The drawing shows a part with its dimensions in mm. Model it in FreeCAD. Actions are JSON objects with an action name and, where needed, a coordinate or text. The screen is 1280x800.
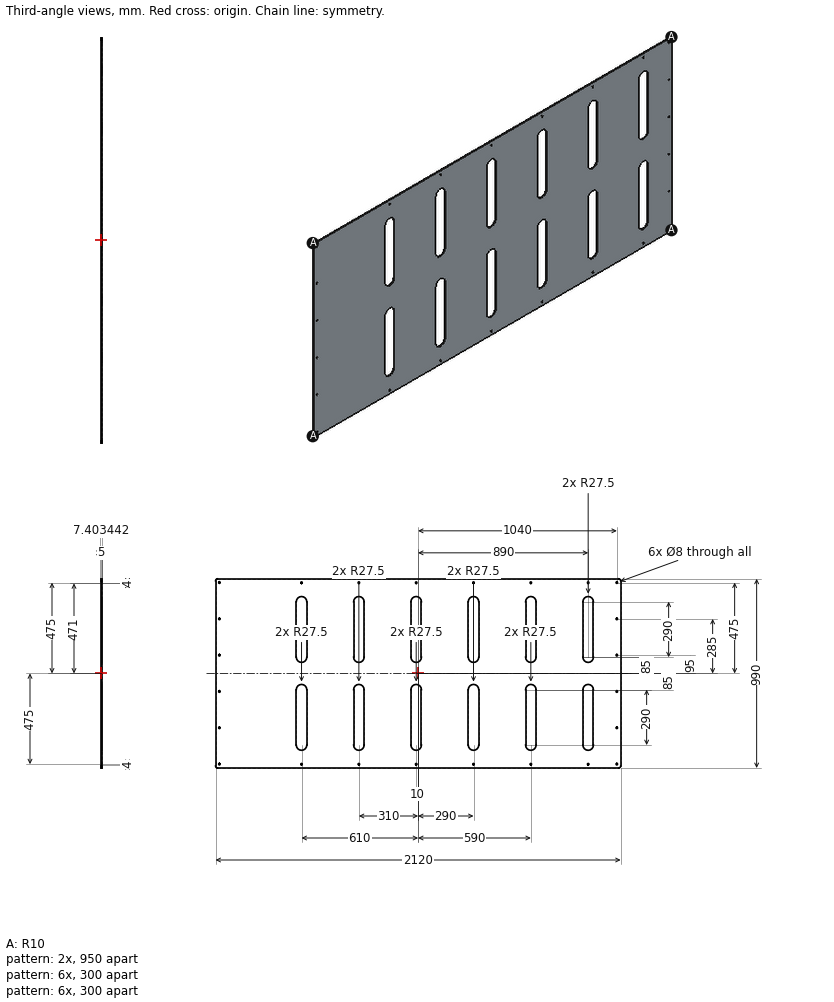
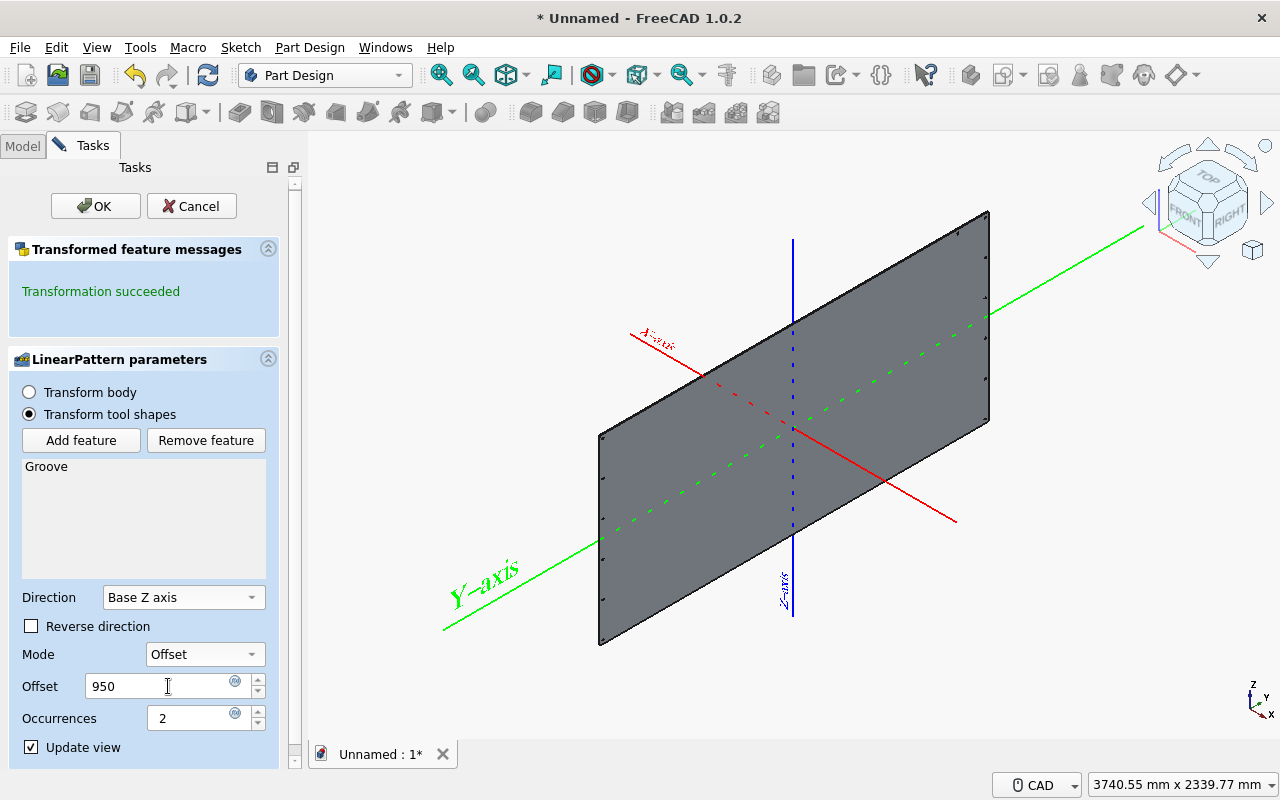
{"action": "triple_click", "coordinate": [198, 718]}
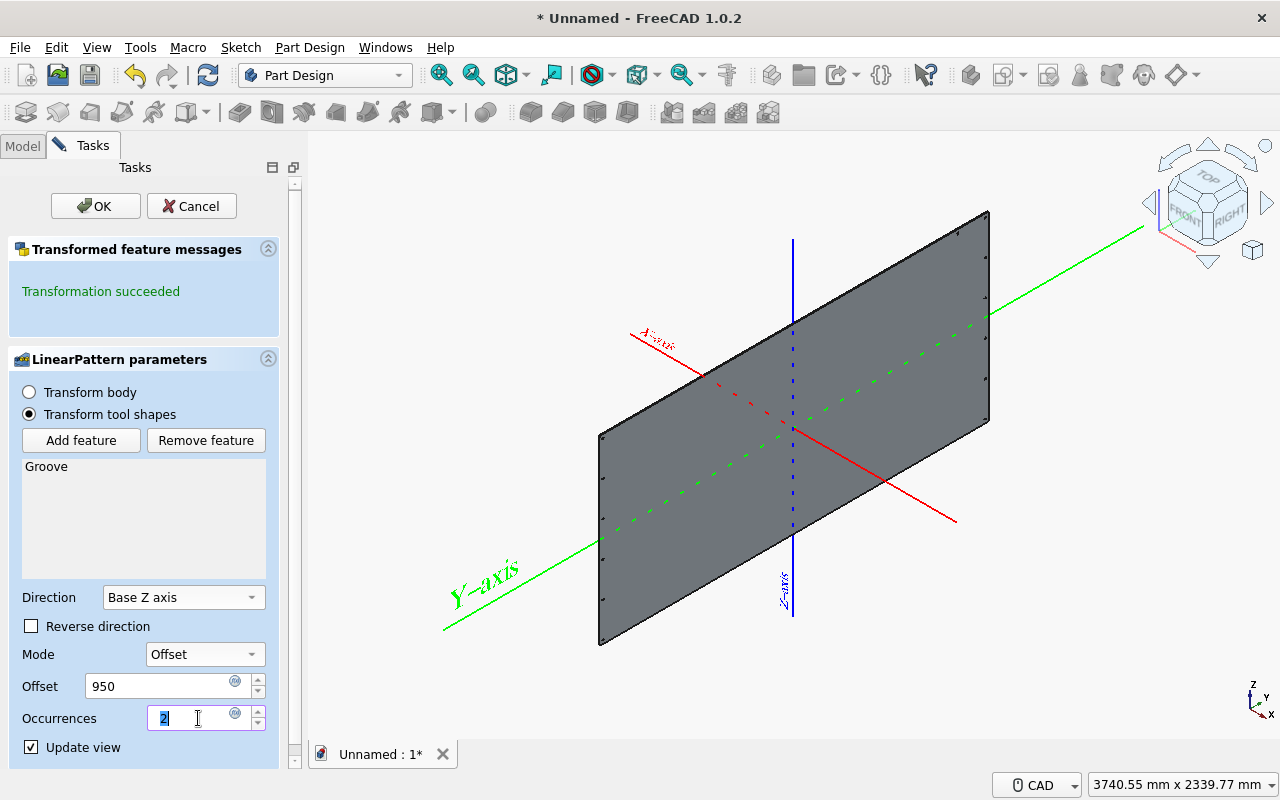
{"action": "type", "text": "2"}
{"action": "key", "text": "Tab"}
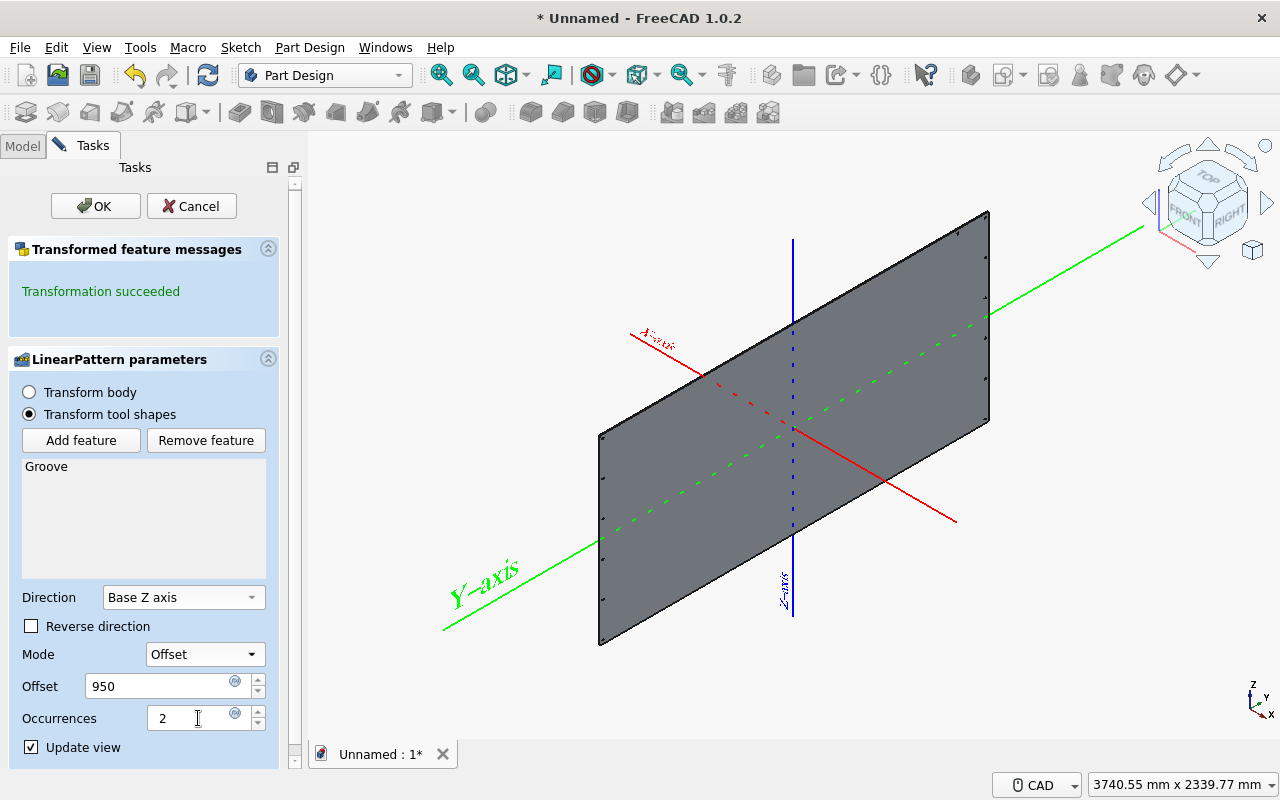
{"action": "left_click", "coordinate": [30, 626]}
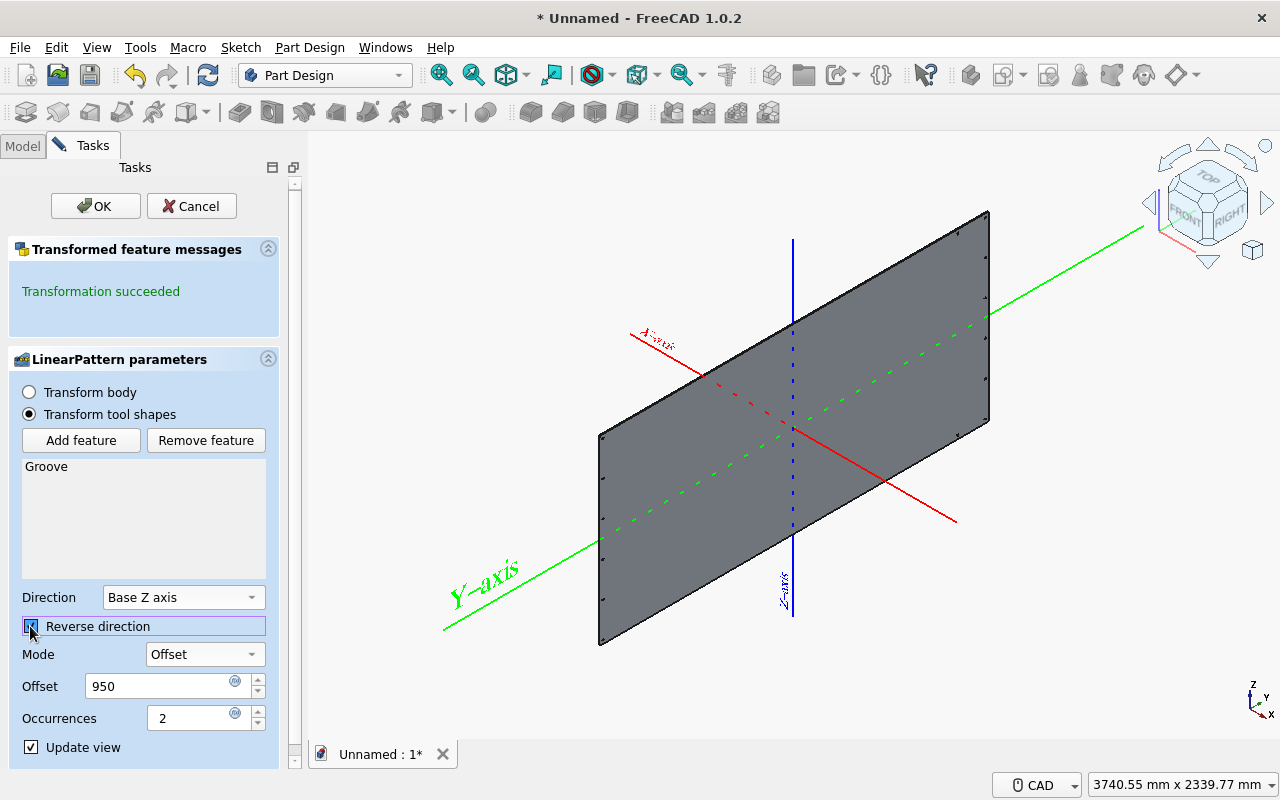
{"action": "left_click", "coordinate": [96, 206]}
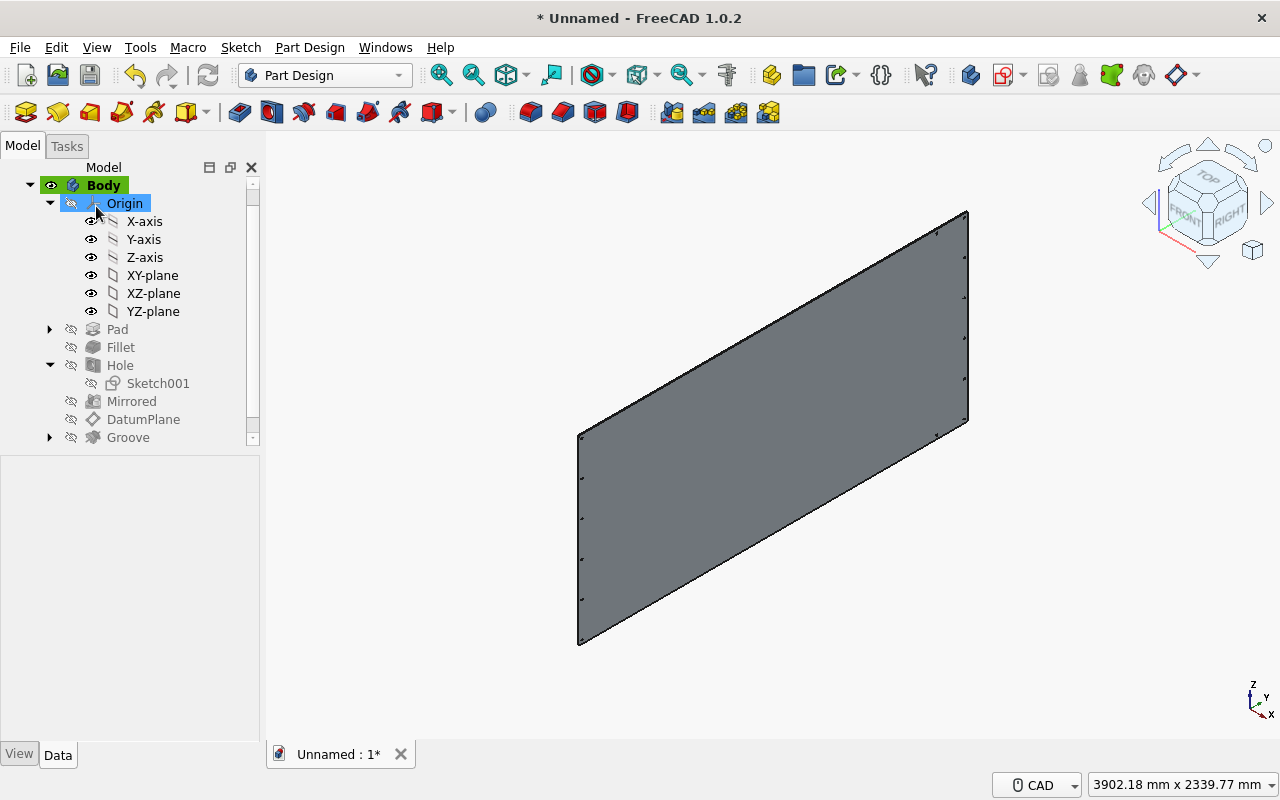
{"action": "left_click", "coordinate": [116, 437]}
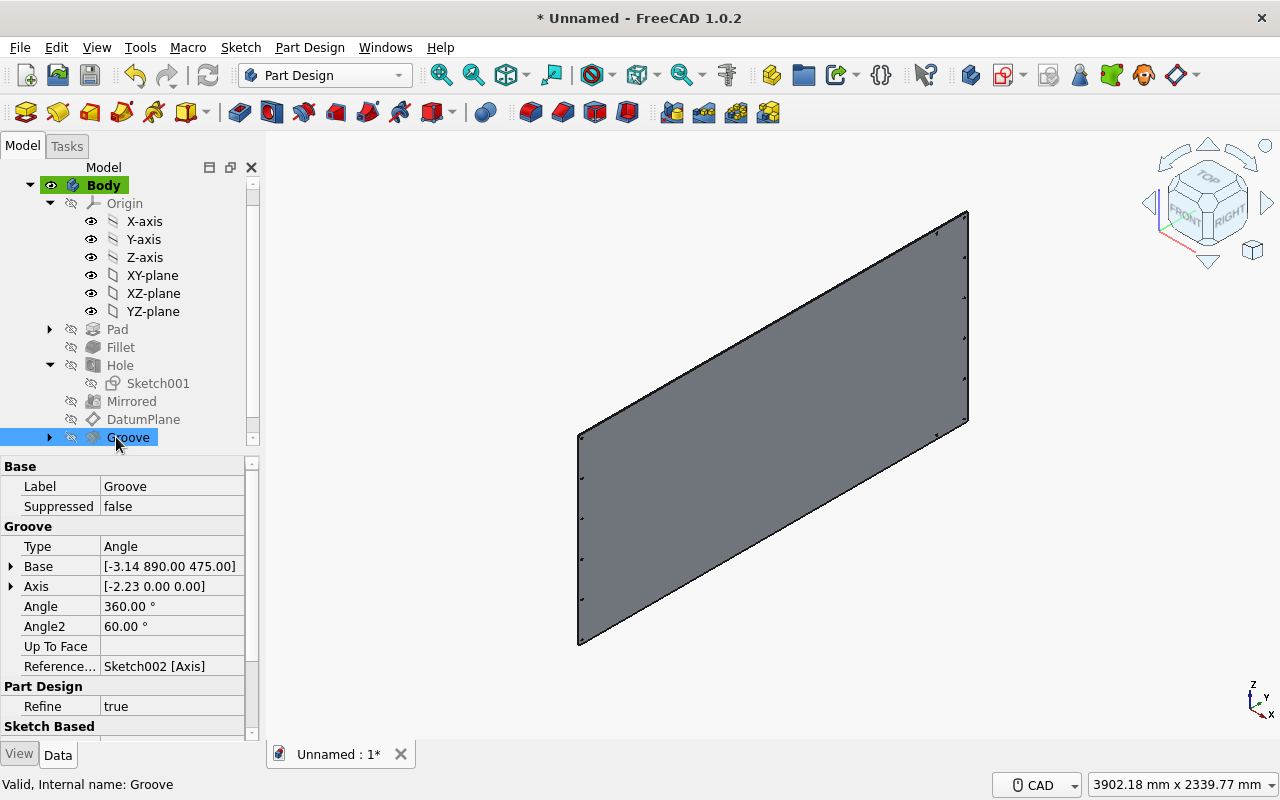
{"action": "left_click", "coordinate": [704, 112]}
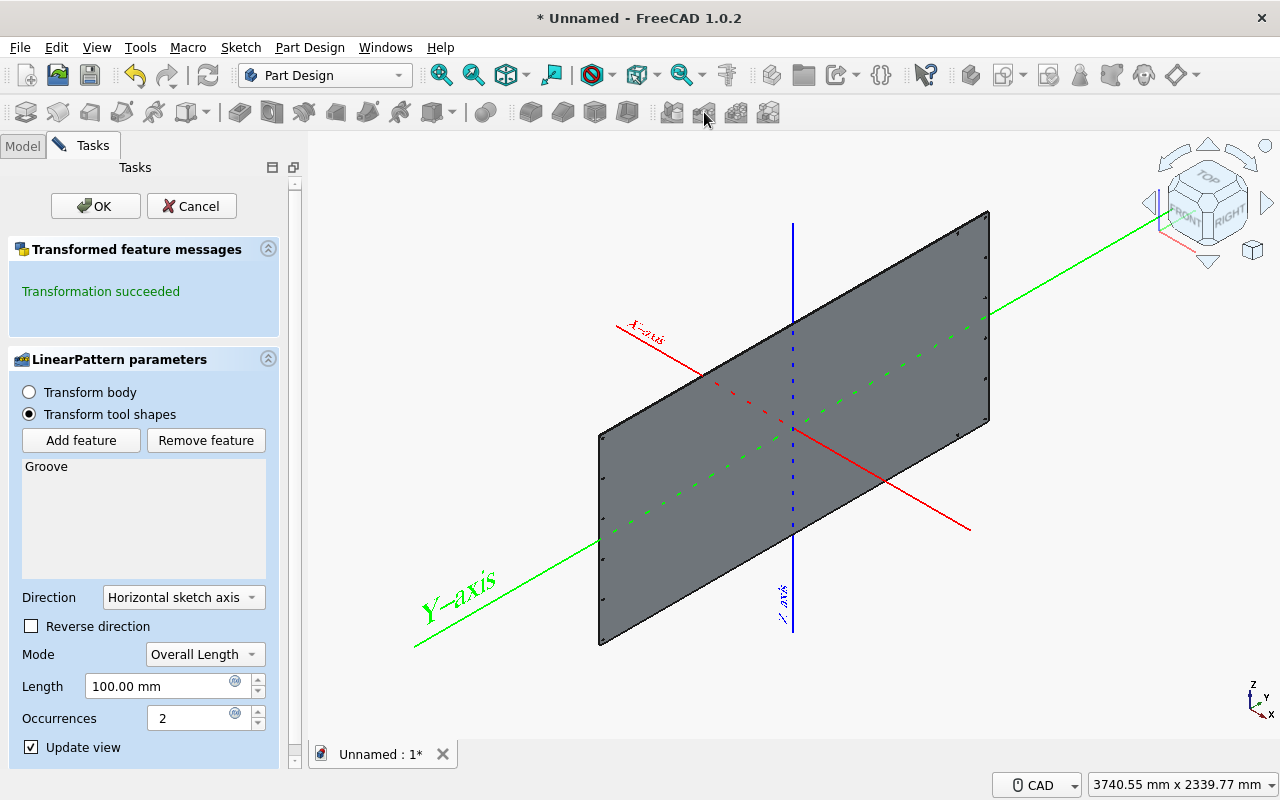
{"action": "left_click", "coordinate": [184, 598]}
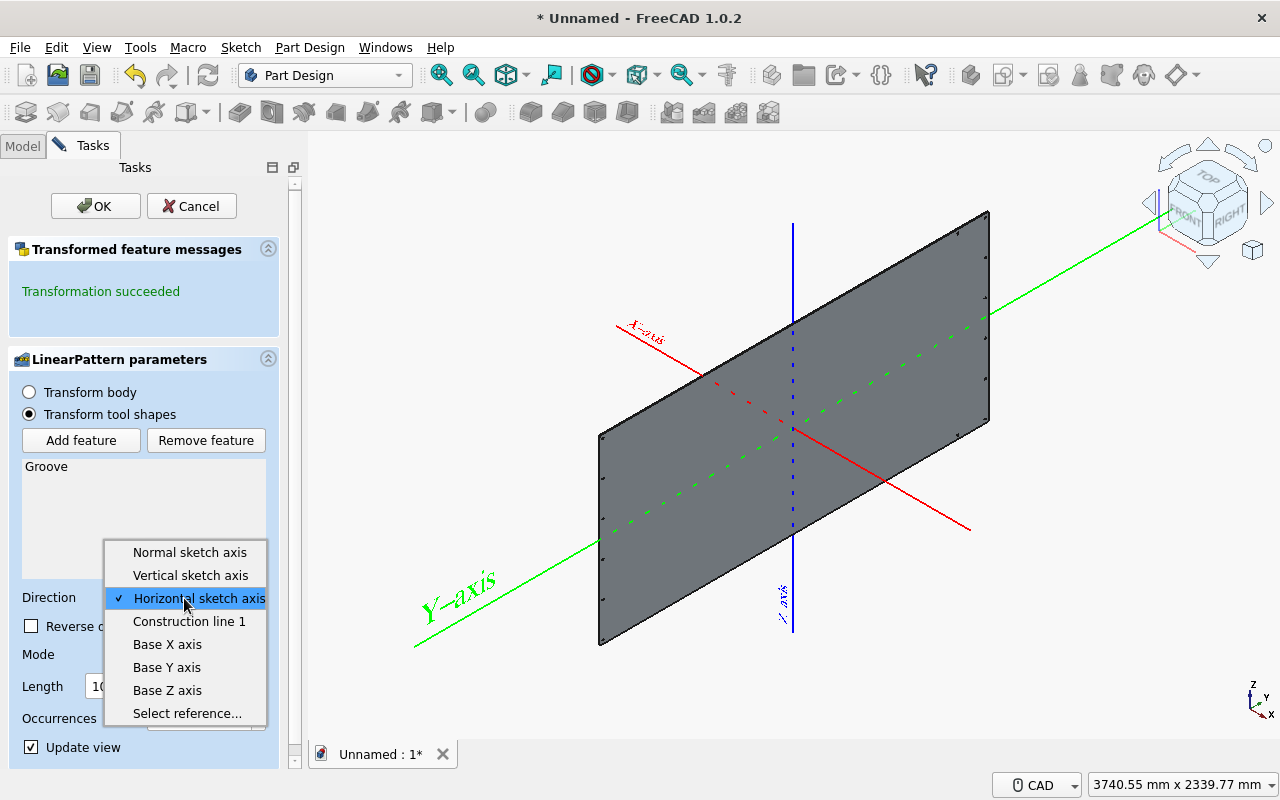
{"action": "left_click", "coordinate": [184, 668]}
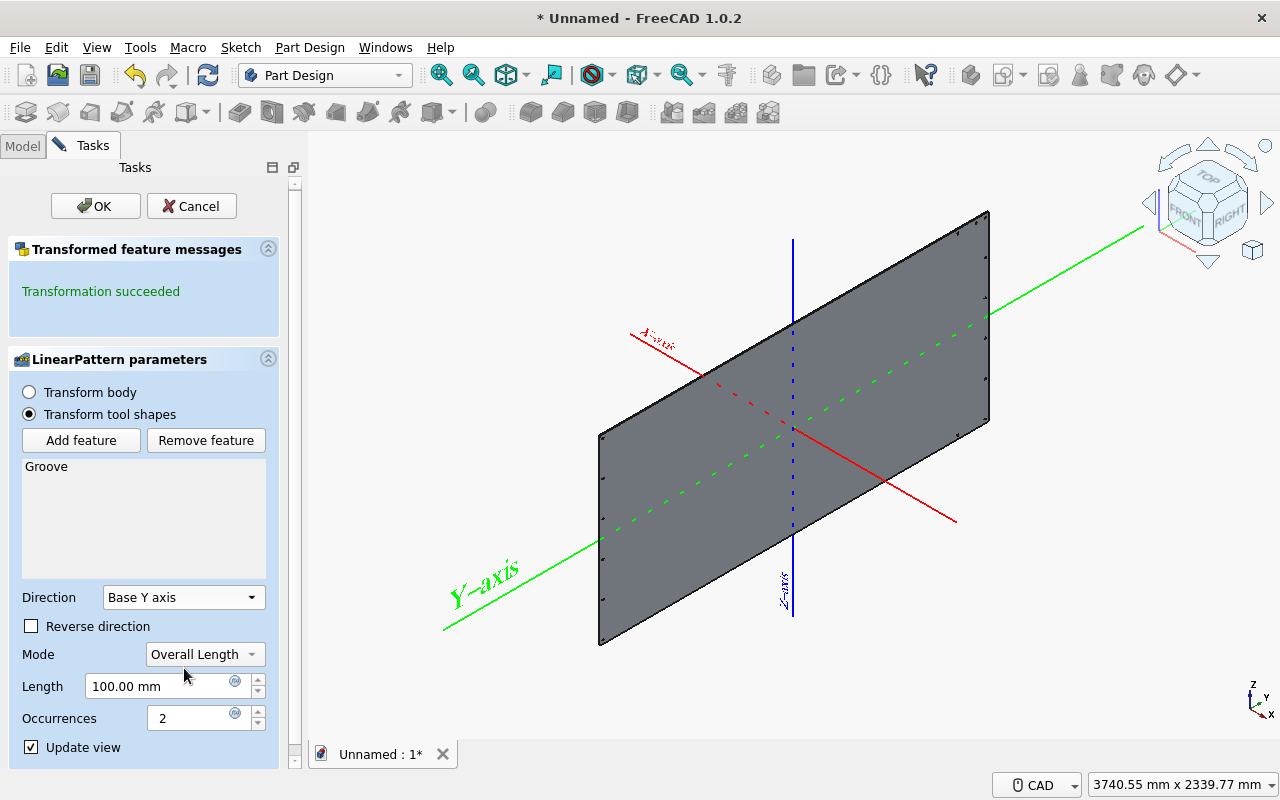
{"action": "left_click", "coordinate": [206, 654]}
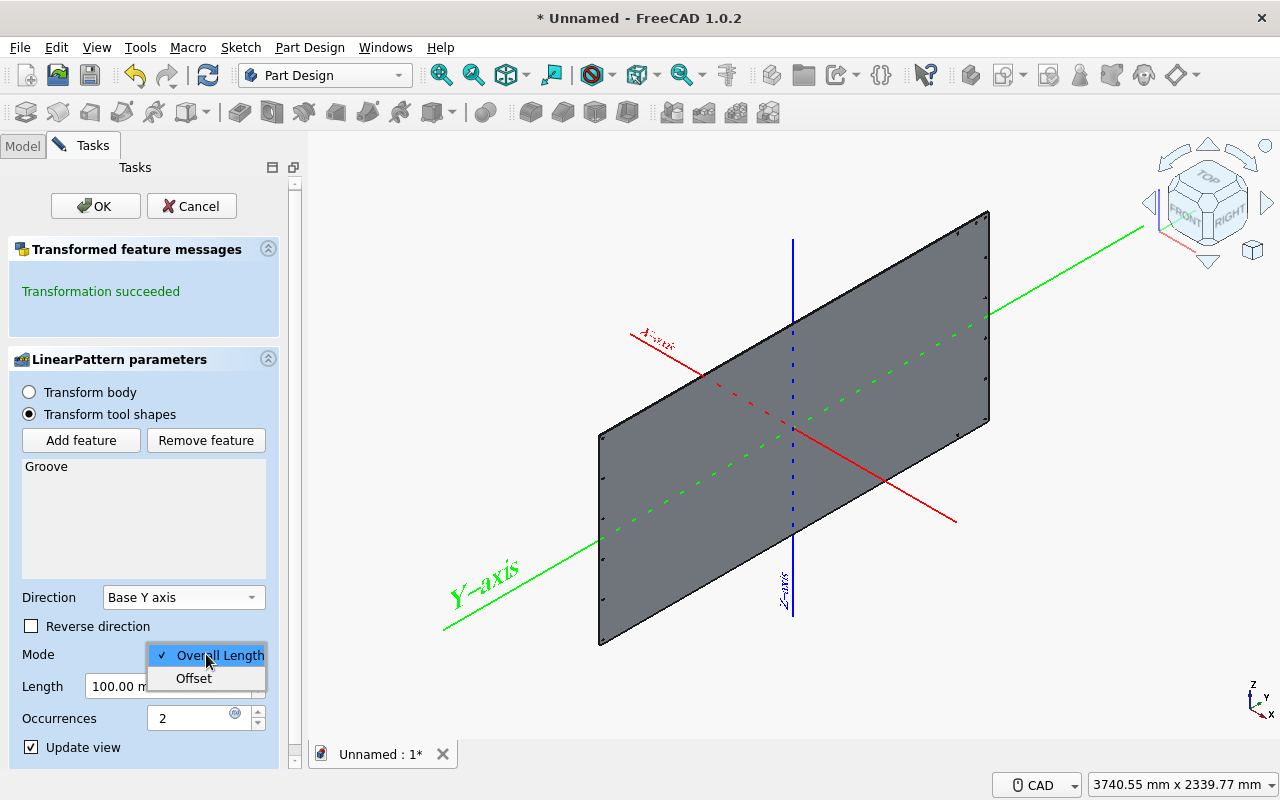
{"action": "left_click", "coordinate": [206, 678]}